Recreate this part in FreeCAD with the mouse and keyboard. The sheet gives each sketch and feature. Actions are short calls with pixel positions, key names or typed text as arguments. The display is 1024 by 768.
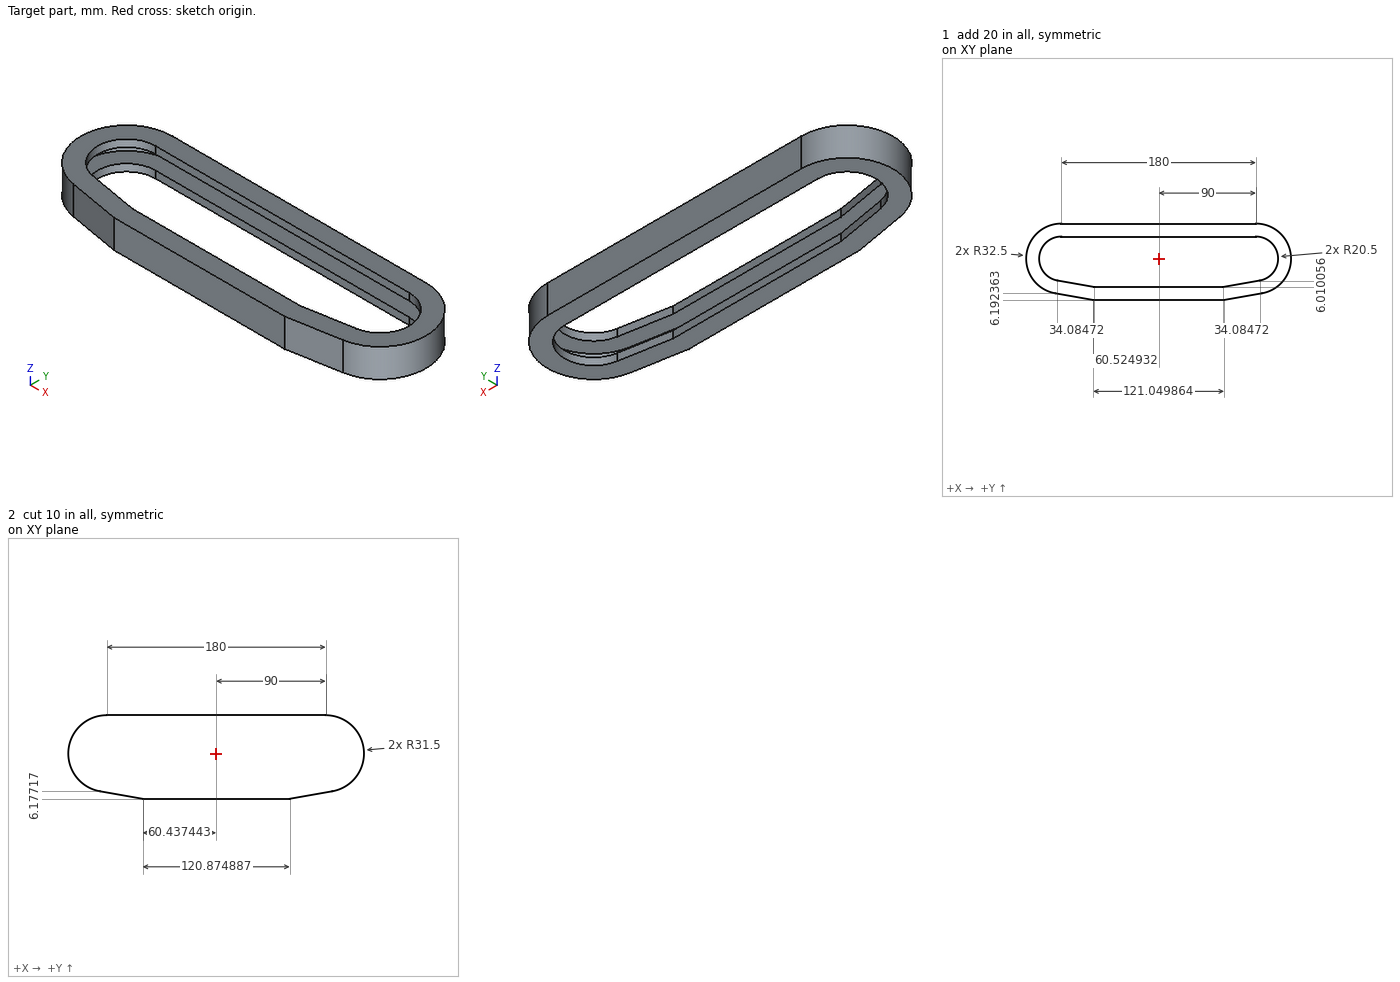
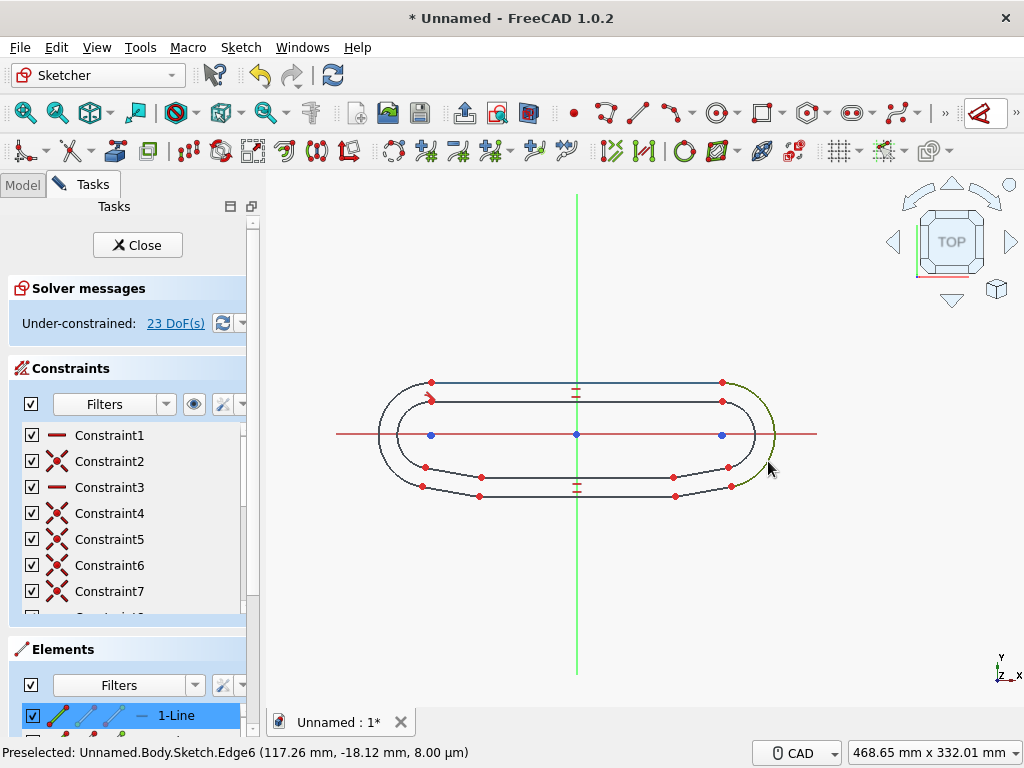
key(t)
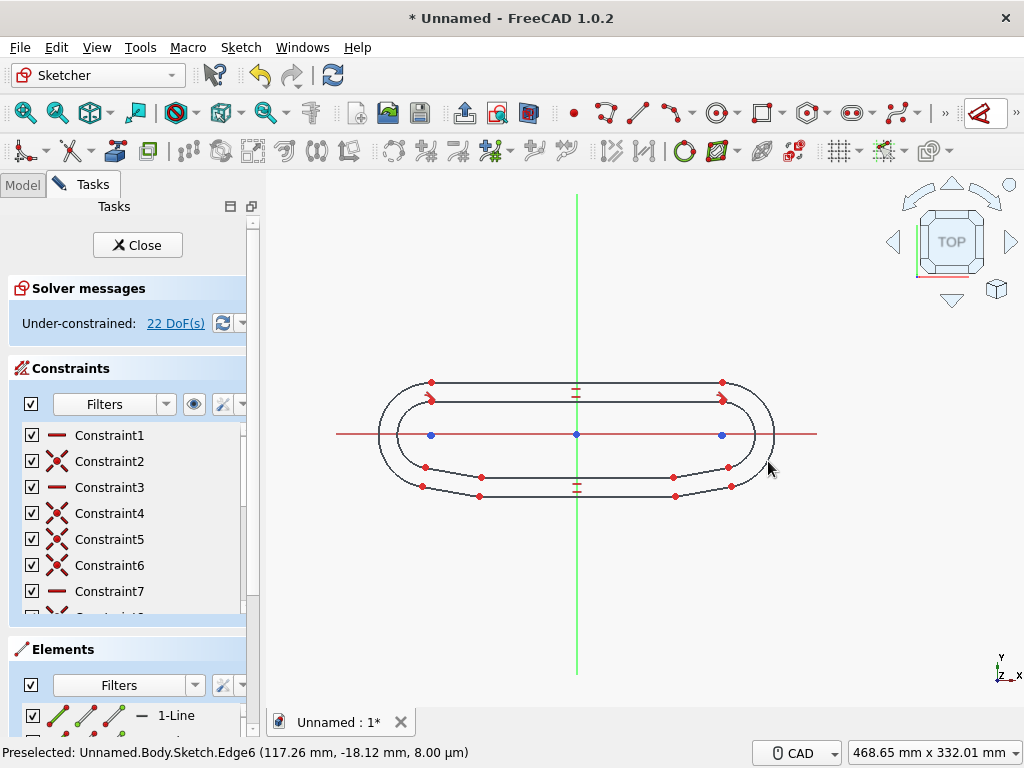
click(439, 490)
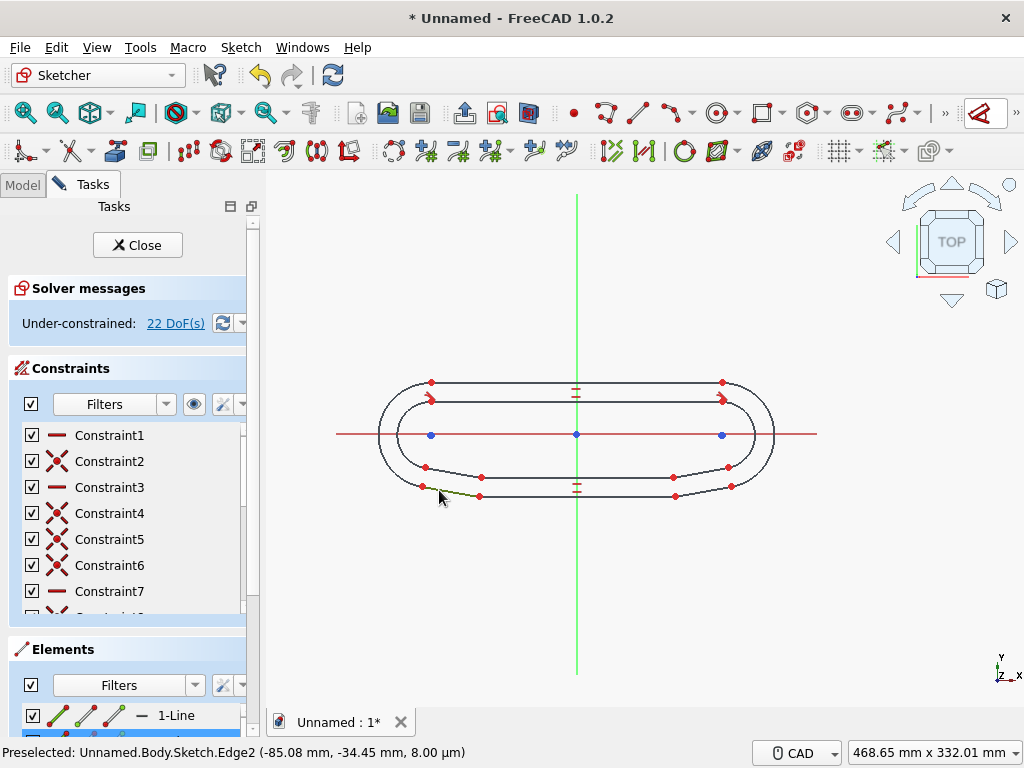
click(390, 402)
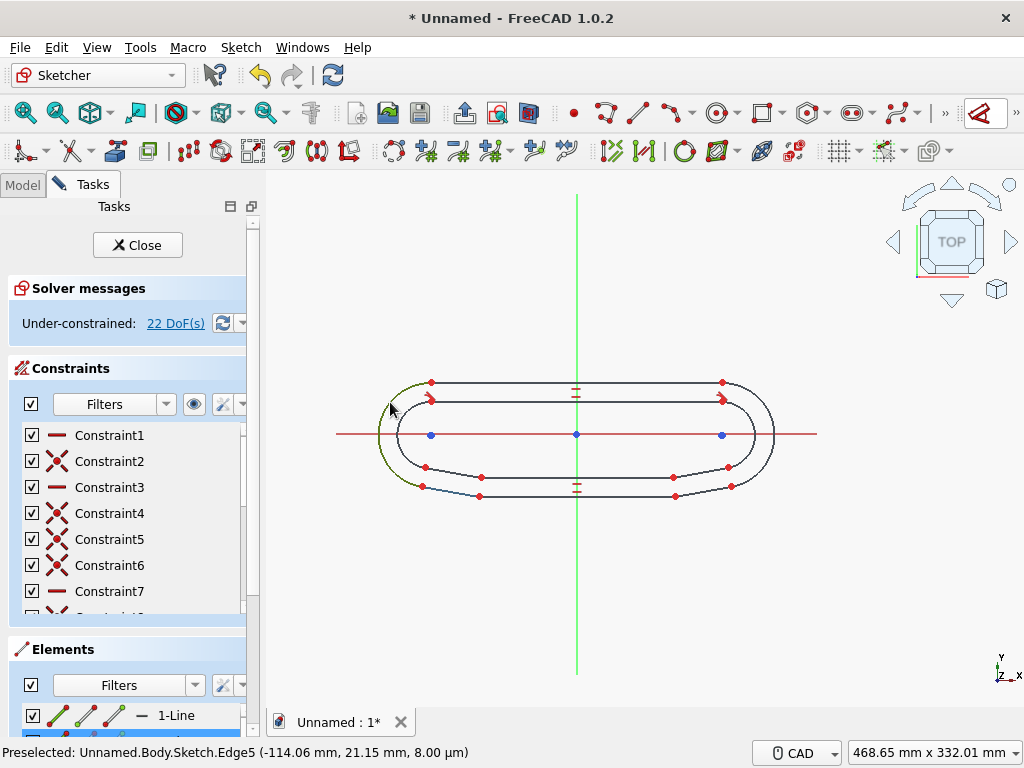
key(t)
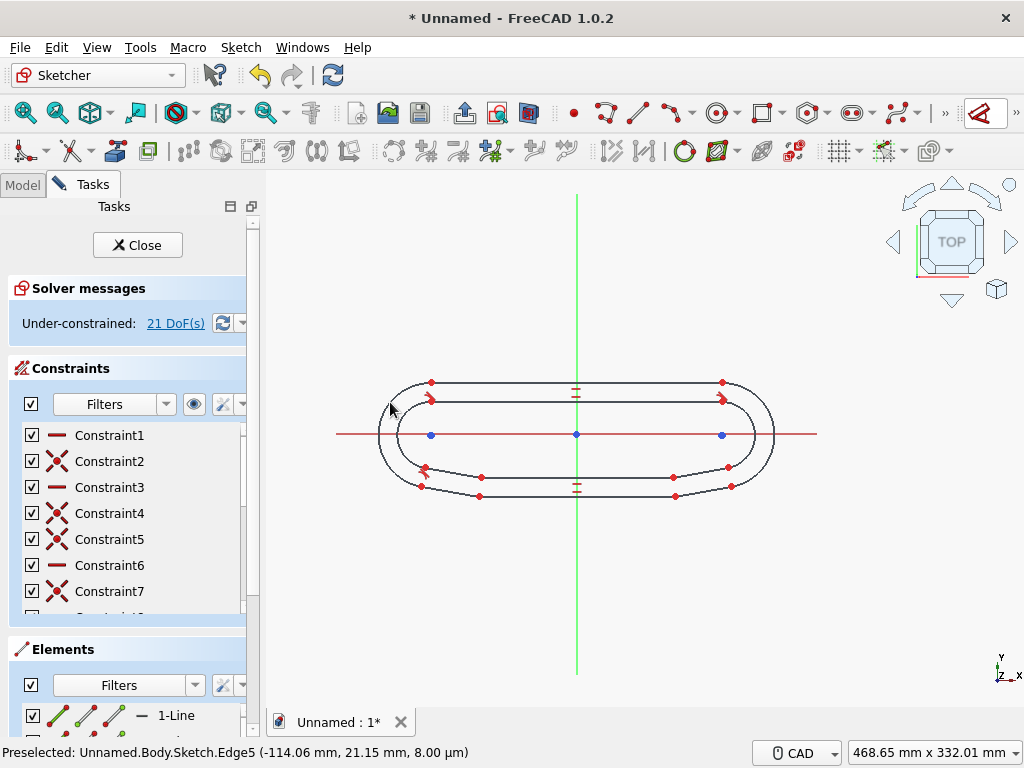
click(692, 494)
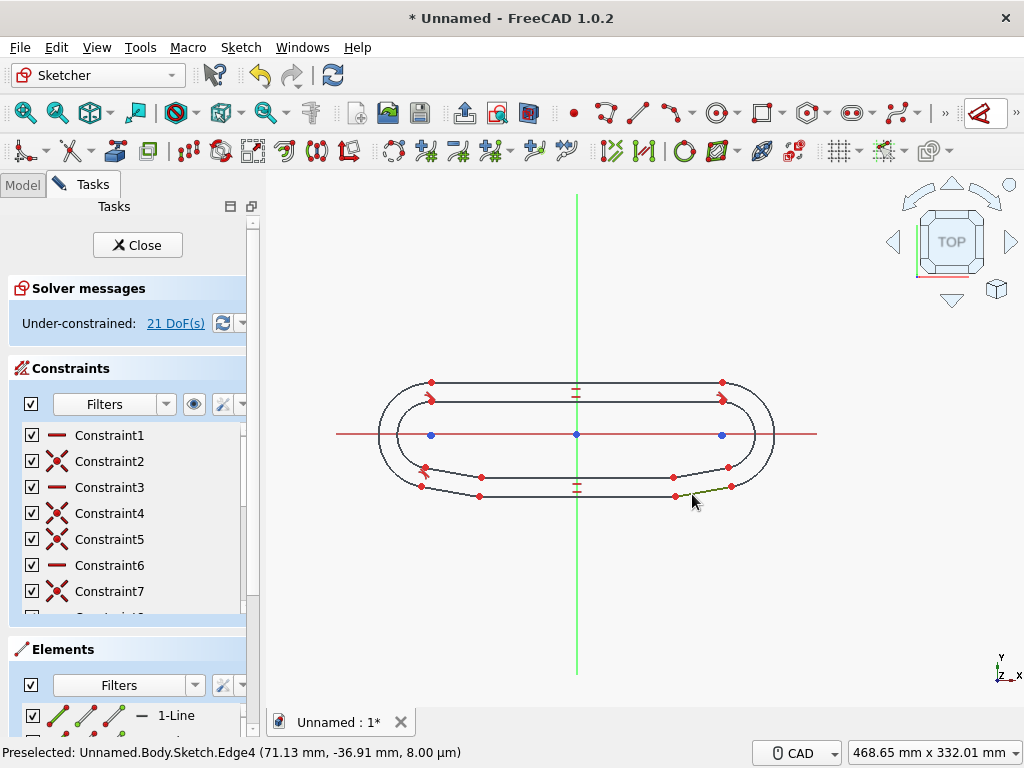
click(768, 461)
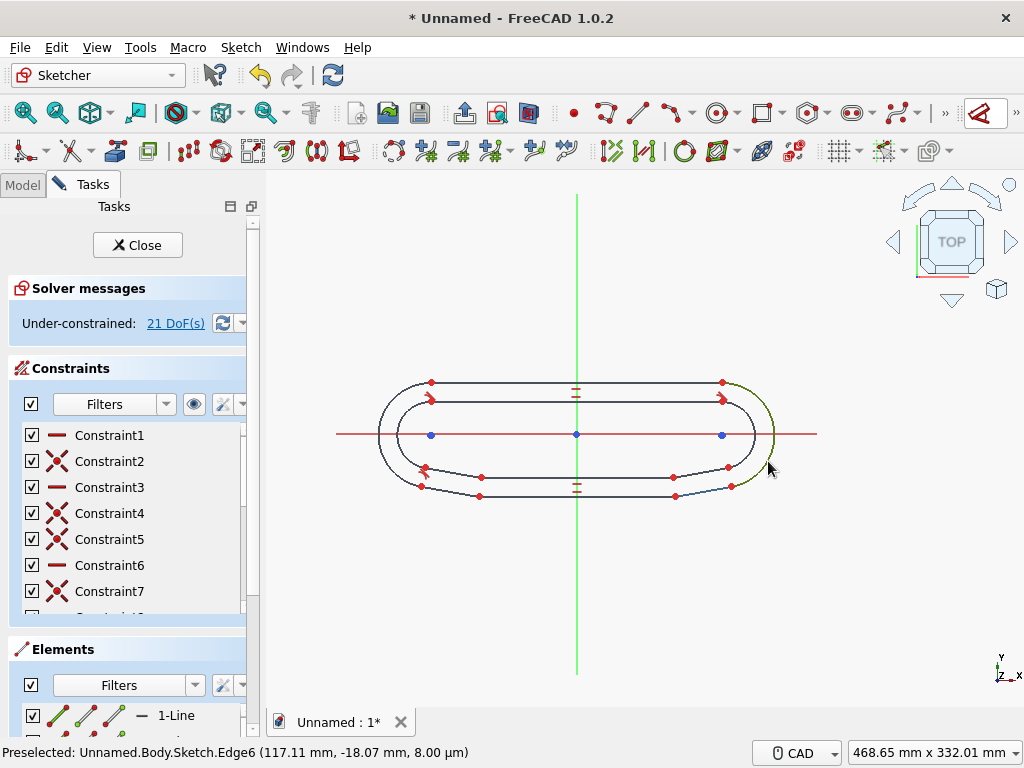
key(t)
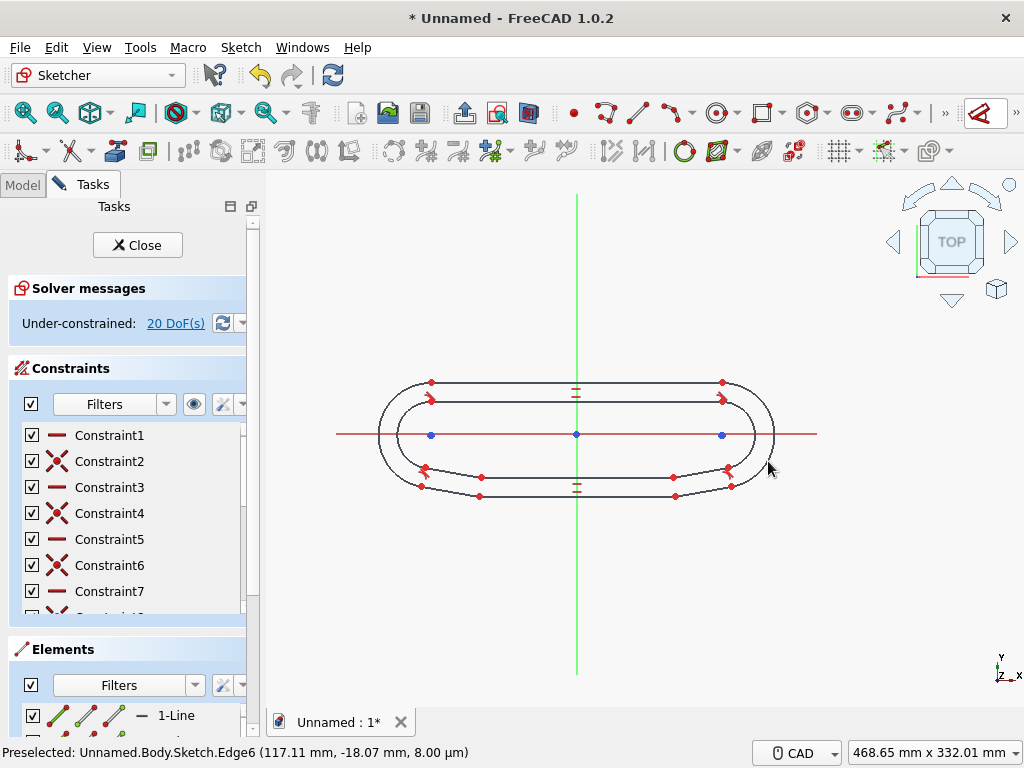
click(518, 402)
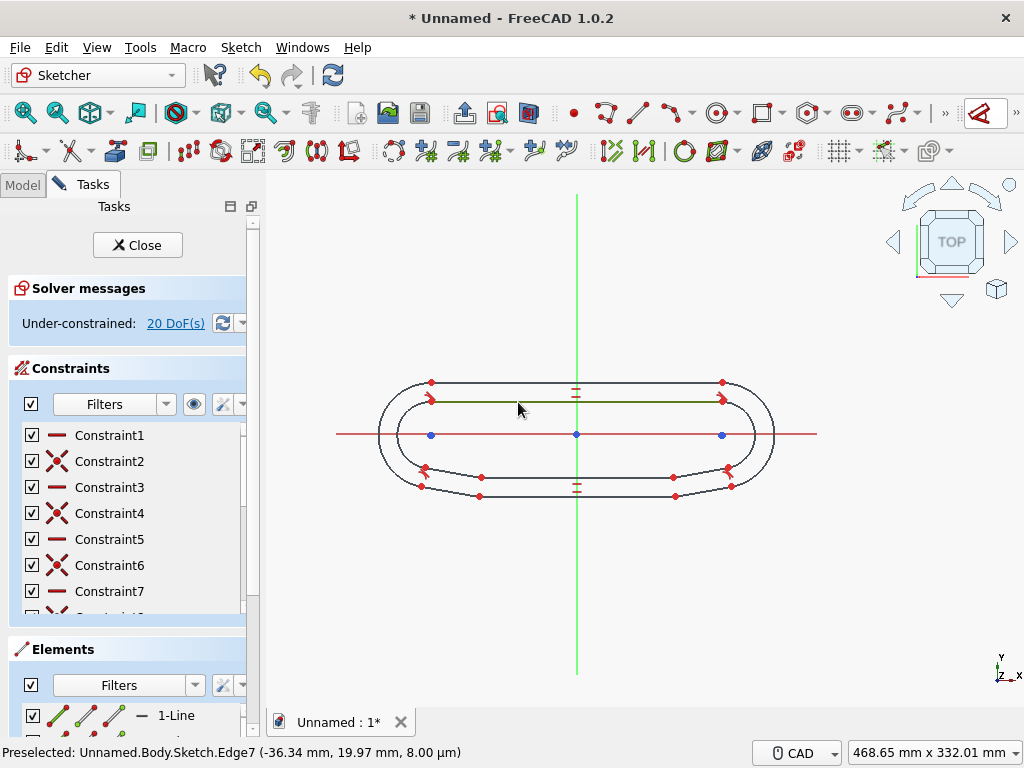
click(751, 451)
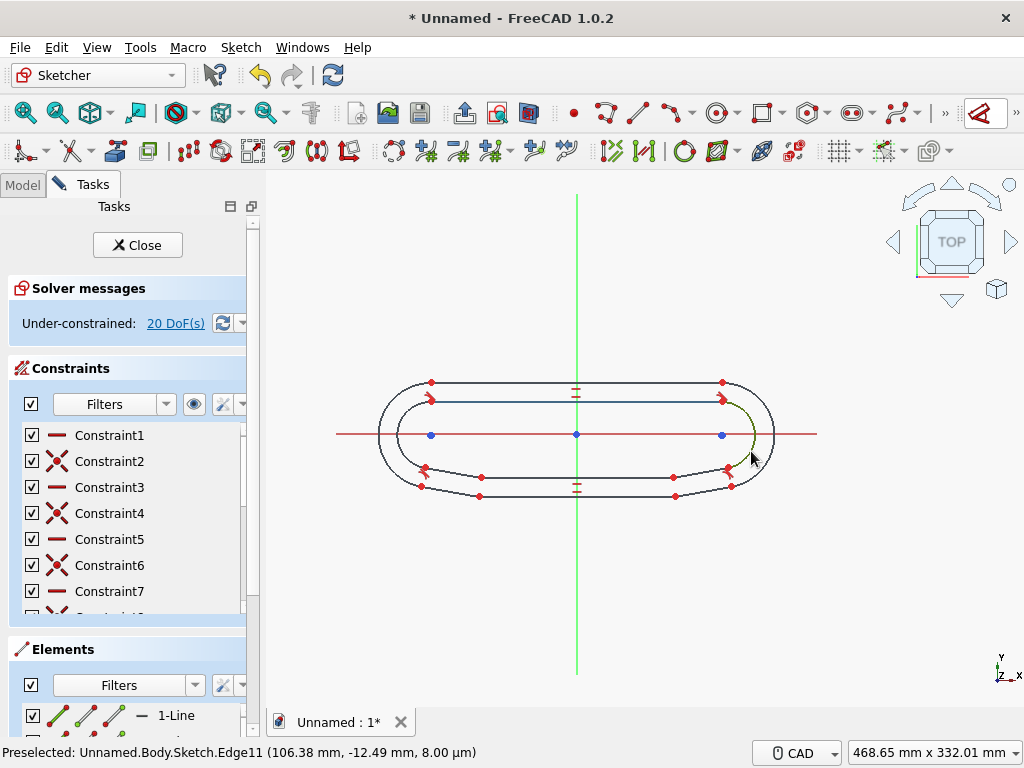
key(t)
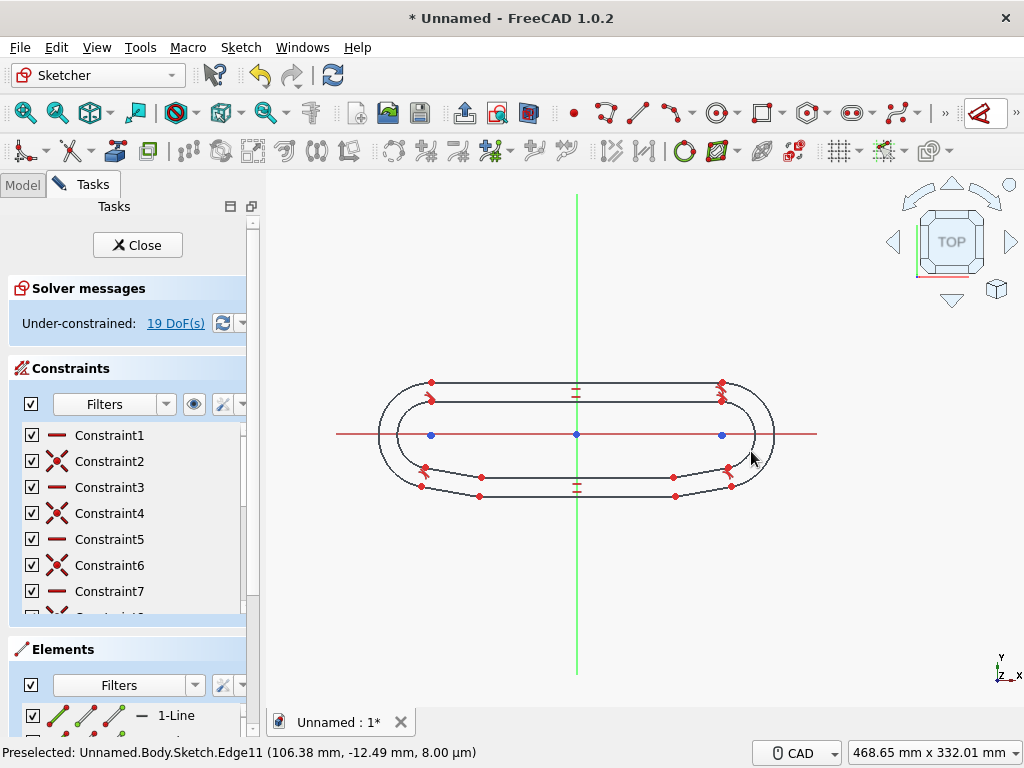
click(518, 402)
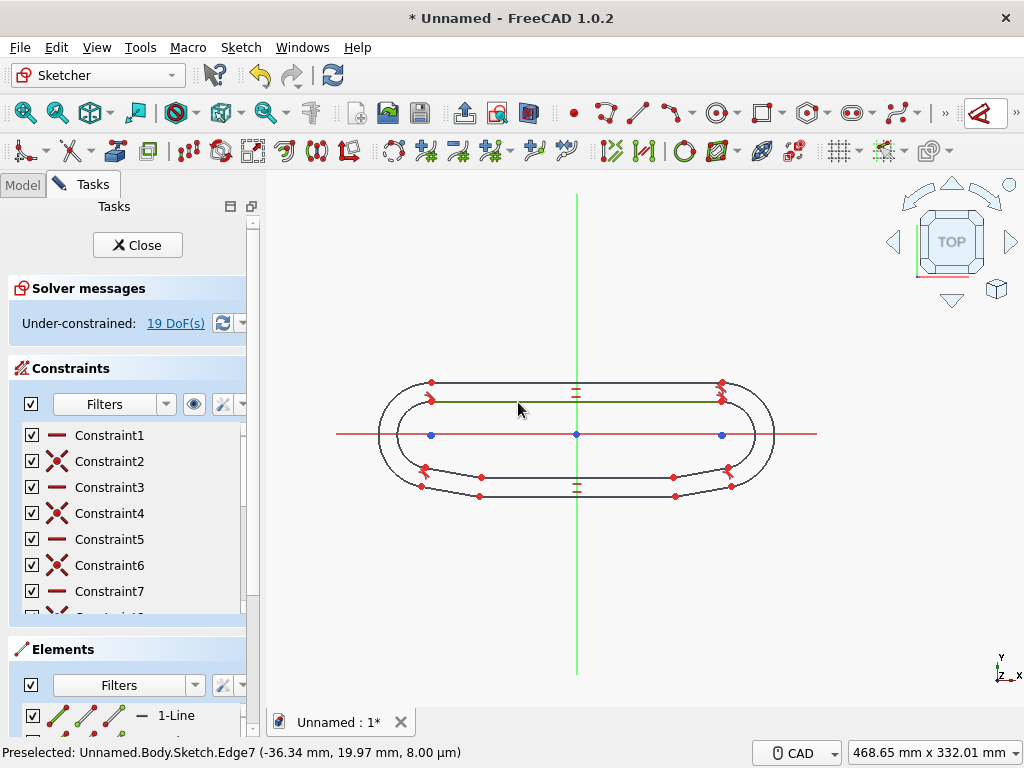
click(405, 414)